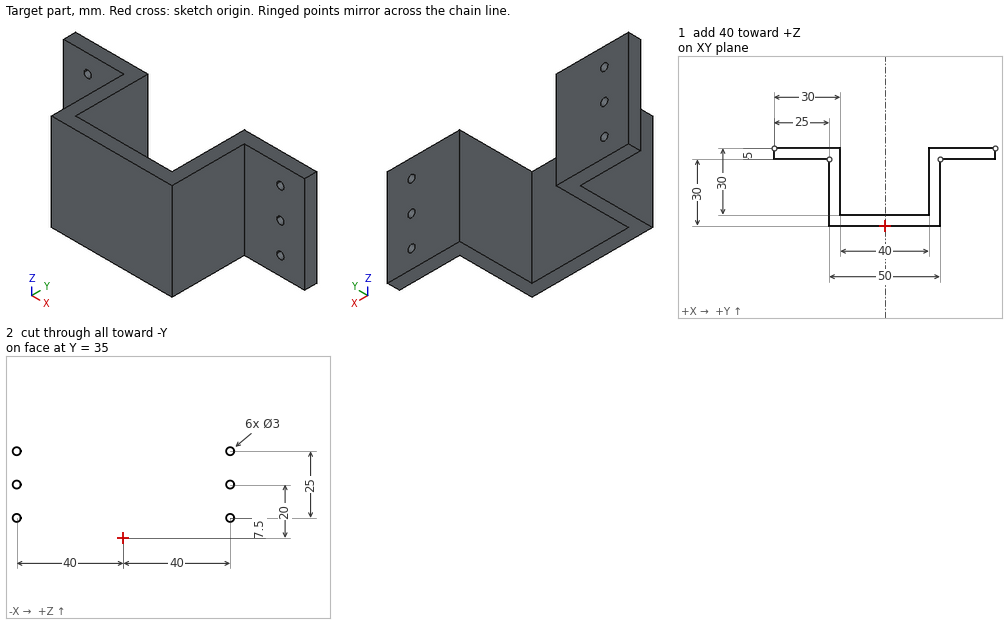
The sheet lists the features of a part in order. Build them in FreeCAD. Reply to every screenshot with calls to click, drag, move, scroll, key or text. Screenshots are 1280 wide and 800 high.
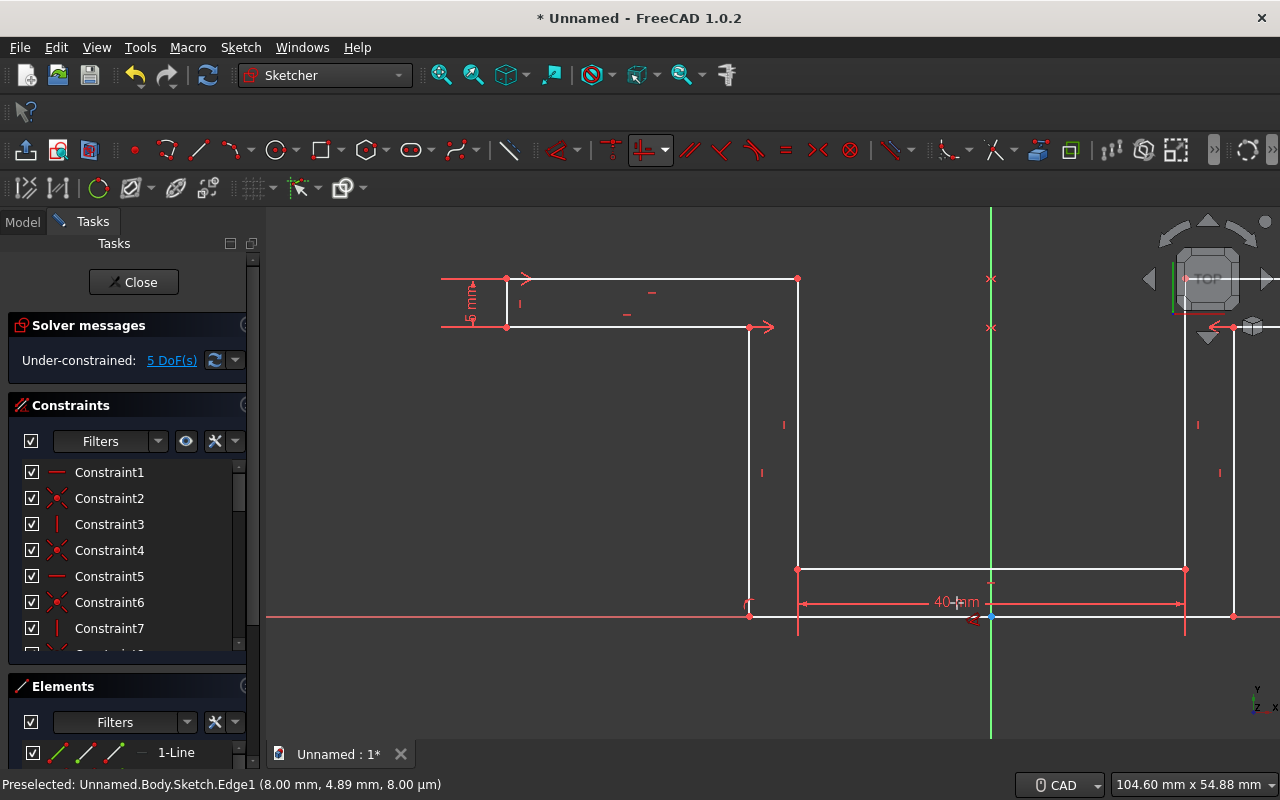
click(798, 482)
click(764, 424)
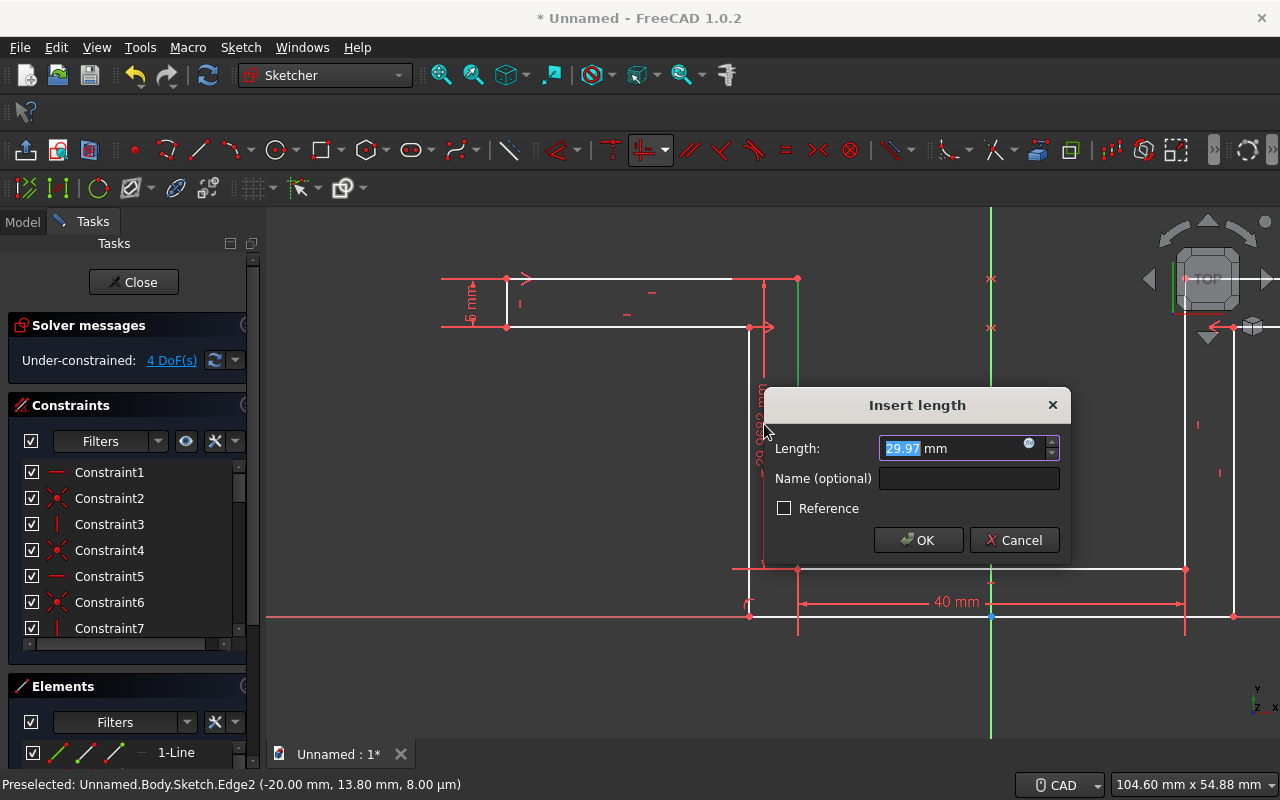
text(30)
key(Return)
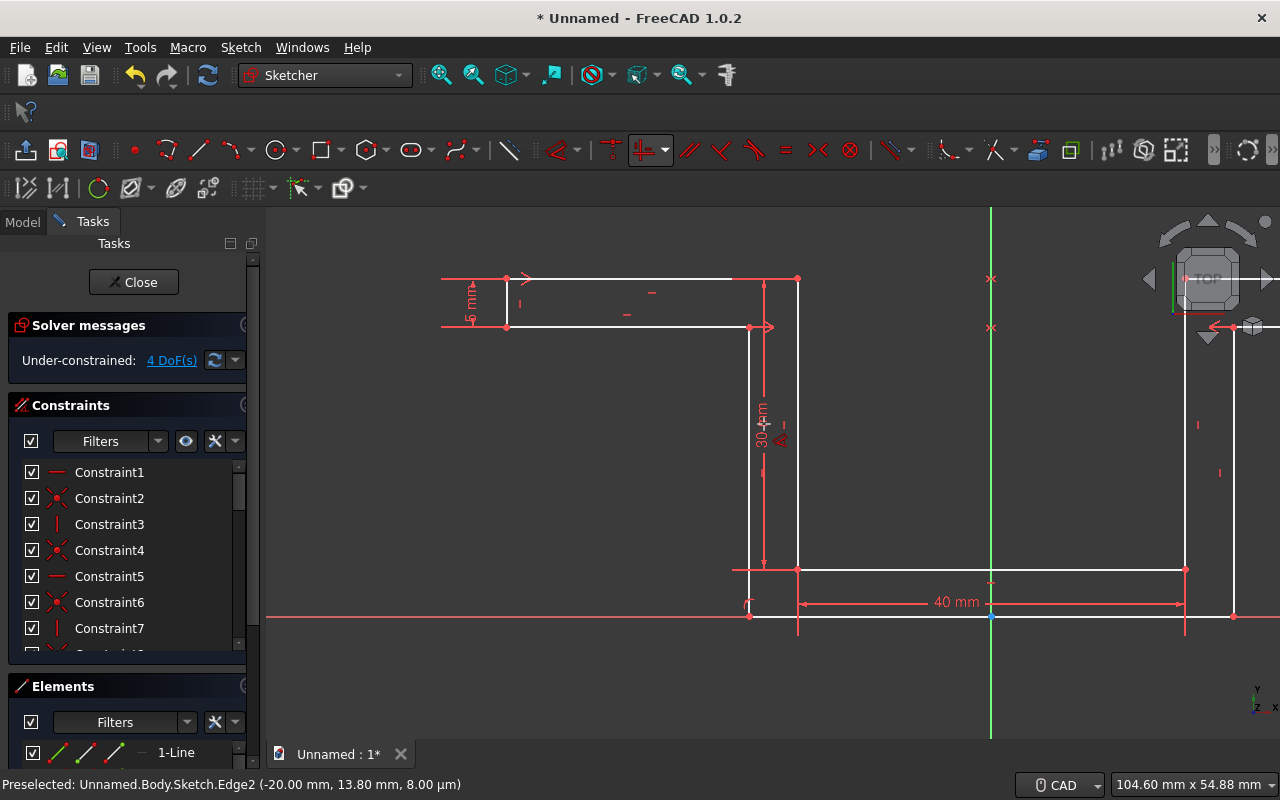
click(710, 279)
click(652, 245)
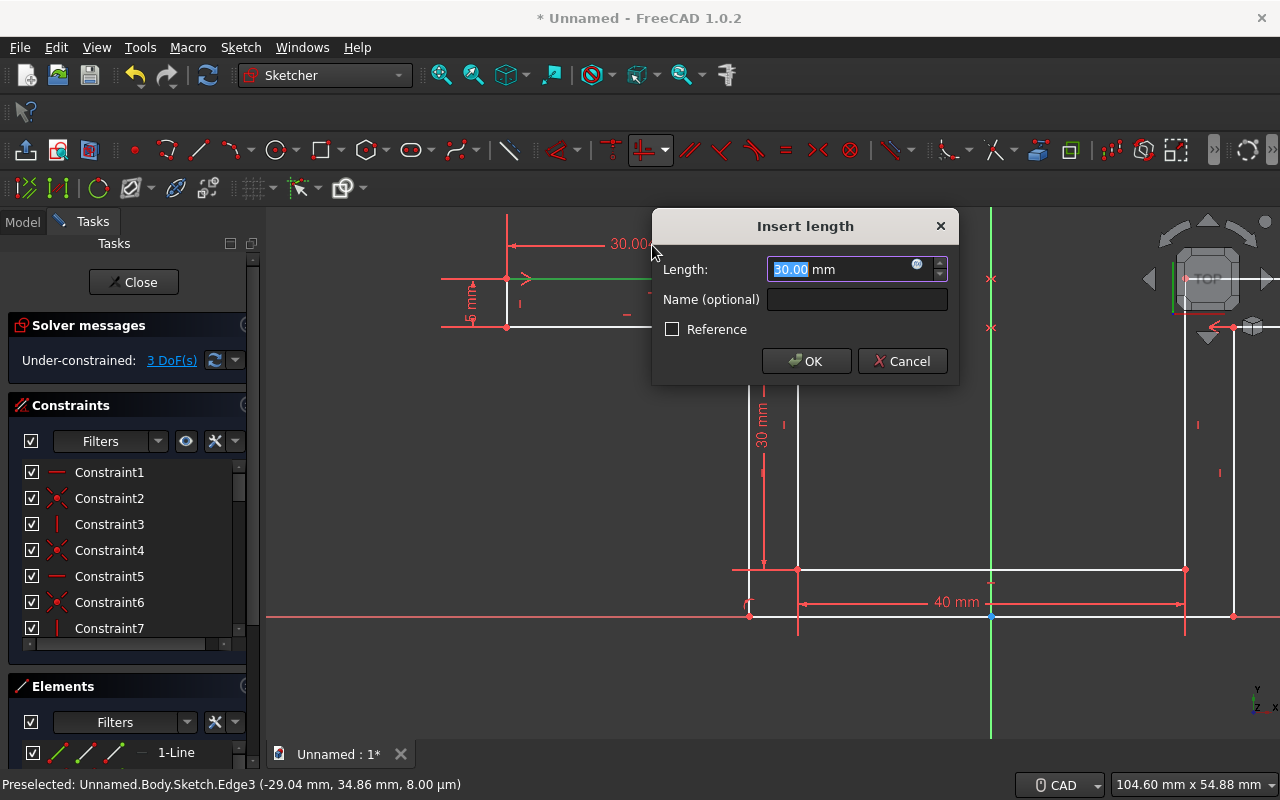
text(30)
key(Return)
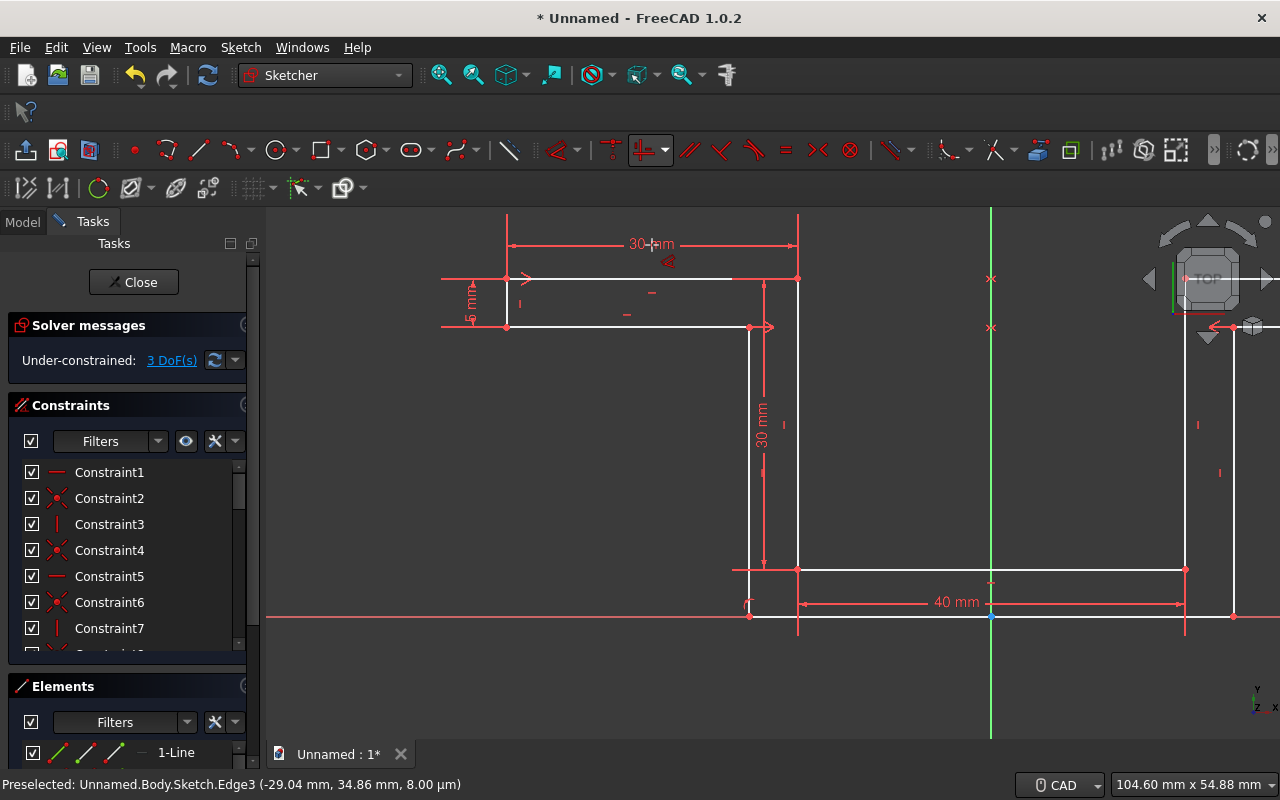
click(580, 327)
click(628, 293)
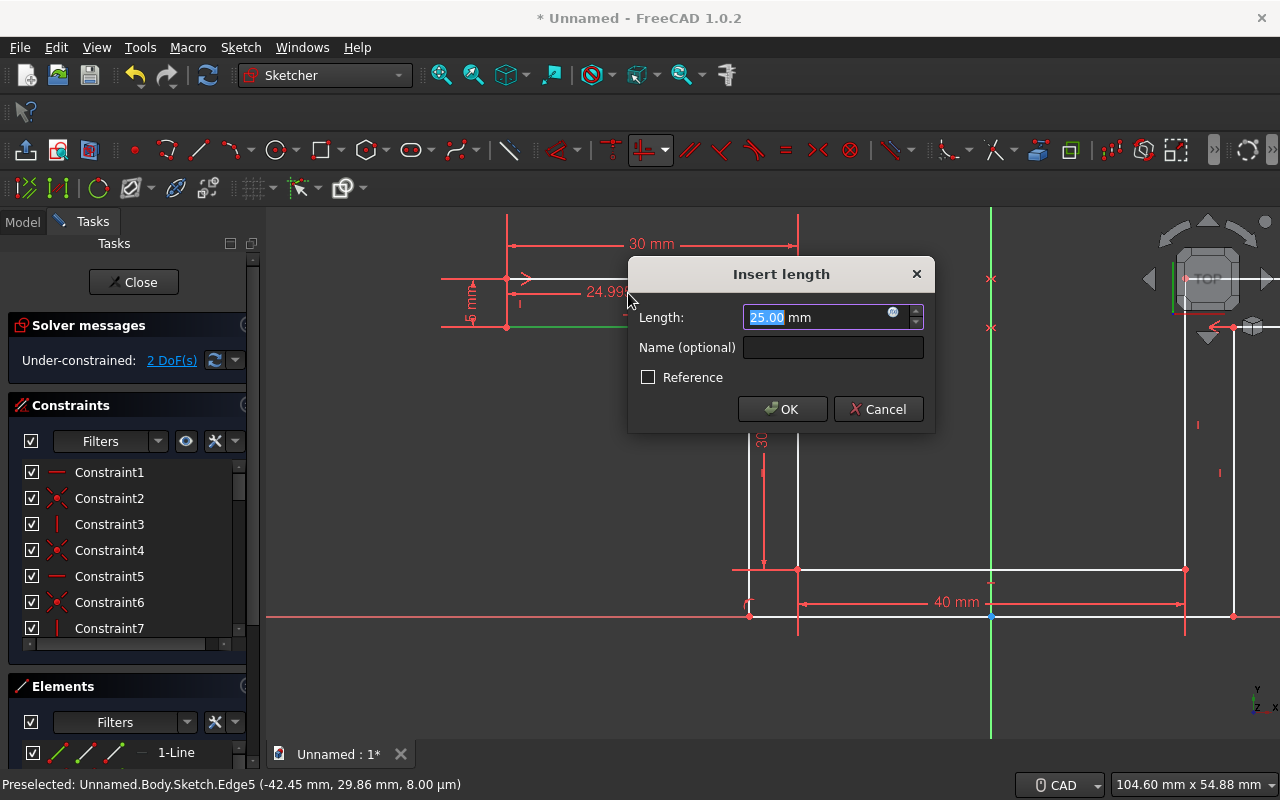
text(25)
key(Return)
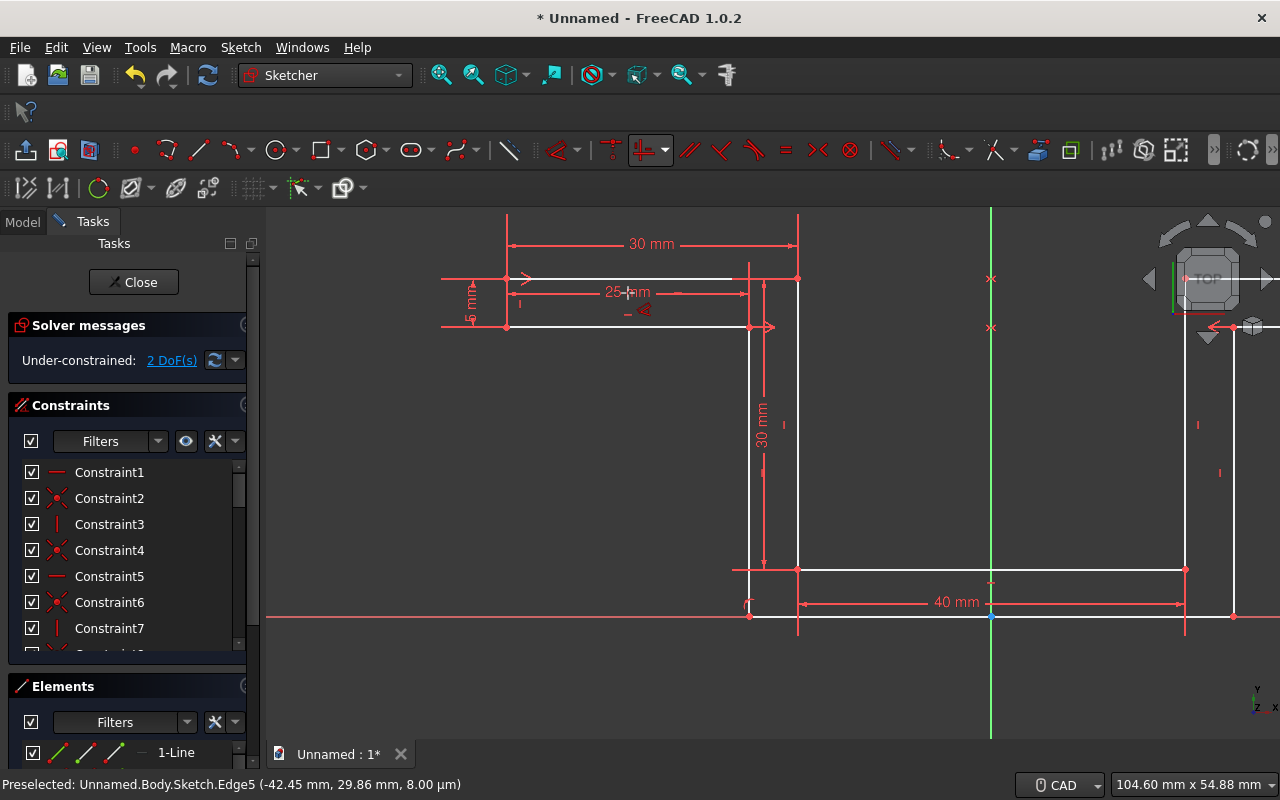
click(749, 414)
click(715, 472)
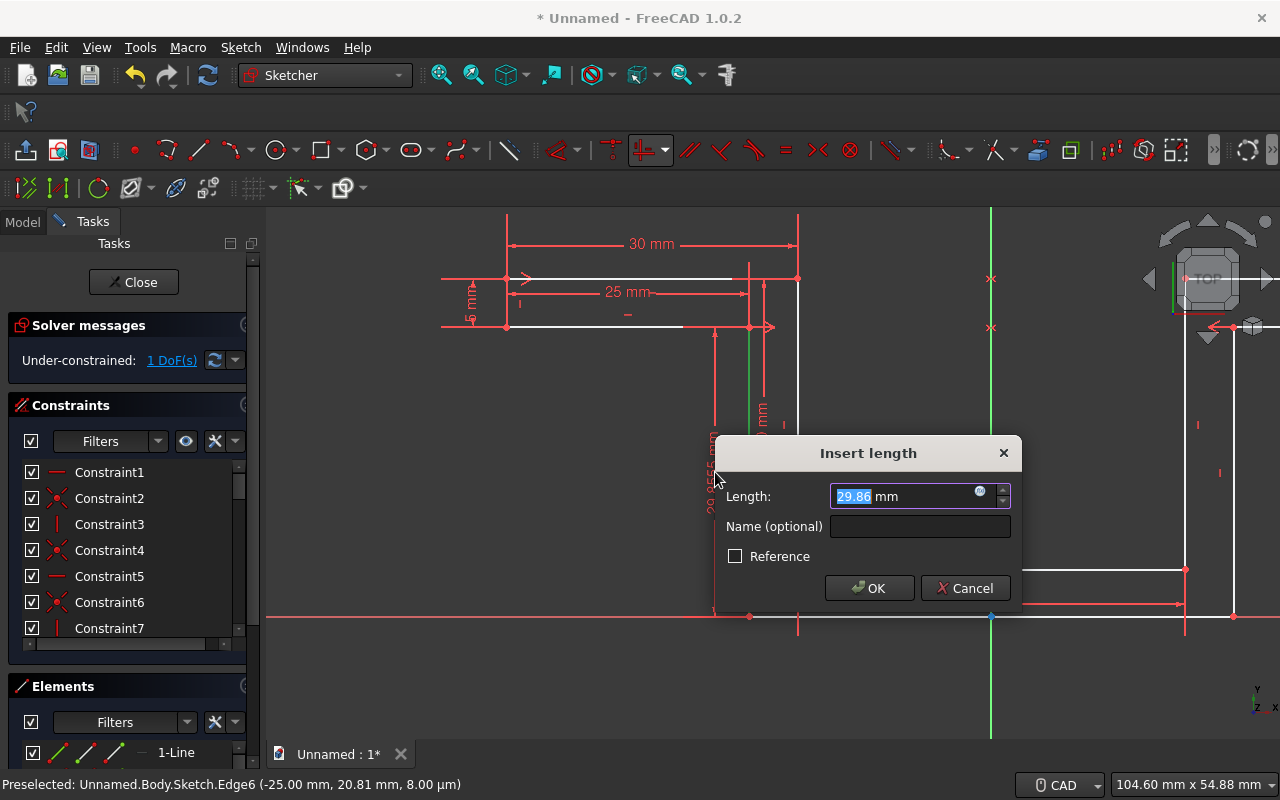
text(30)
key(Return)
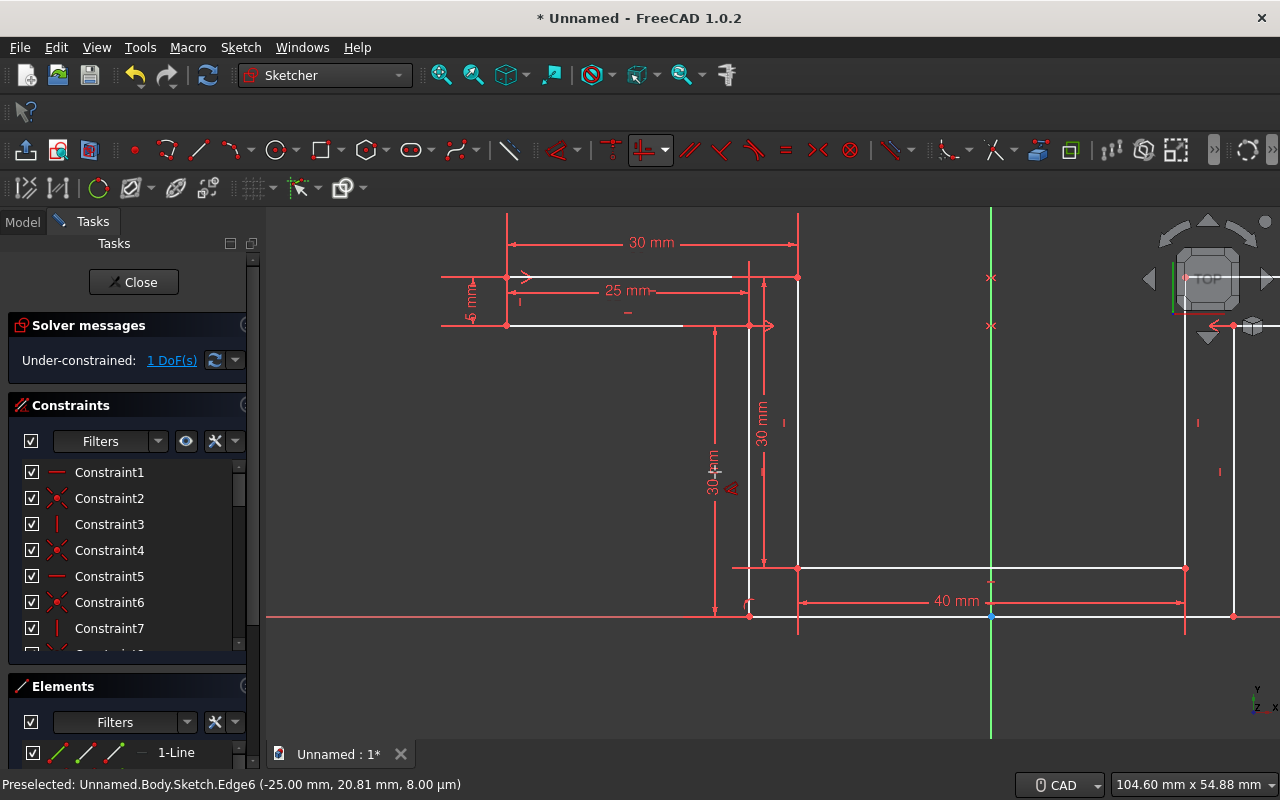
click(895, 617)
click(932, 651)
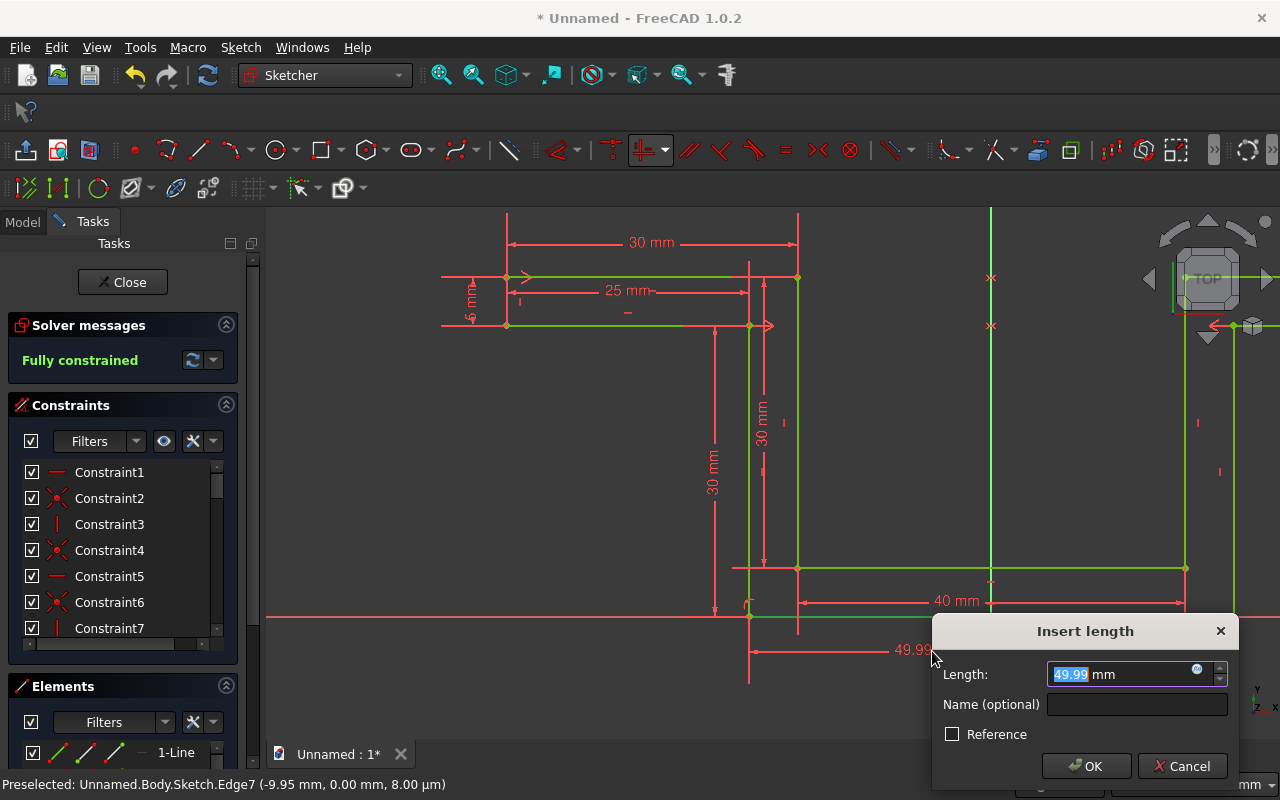
text(50)
key(Return)
key(Escape)